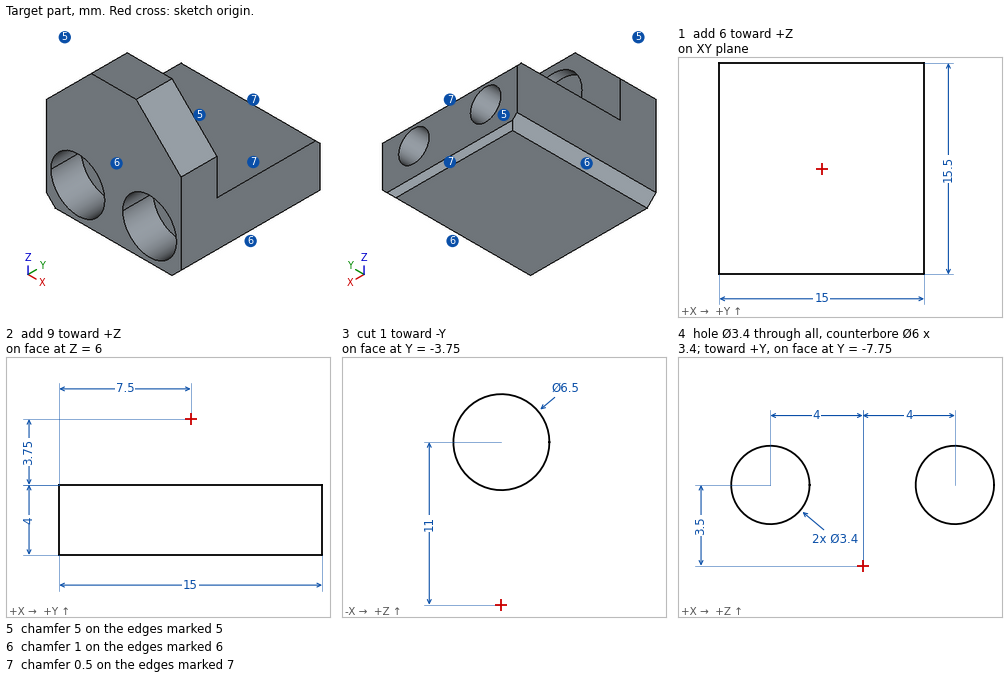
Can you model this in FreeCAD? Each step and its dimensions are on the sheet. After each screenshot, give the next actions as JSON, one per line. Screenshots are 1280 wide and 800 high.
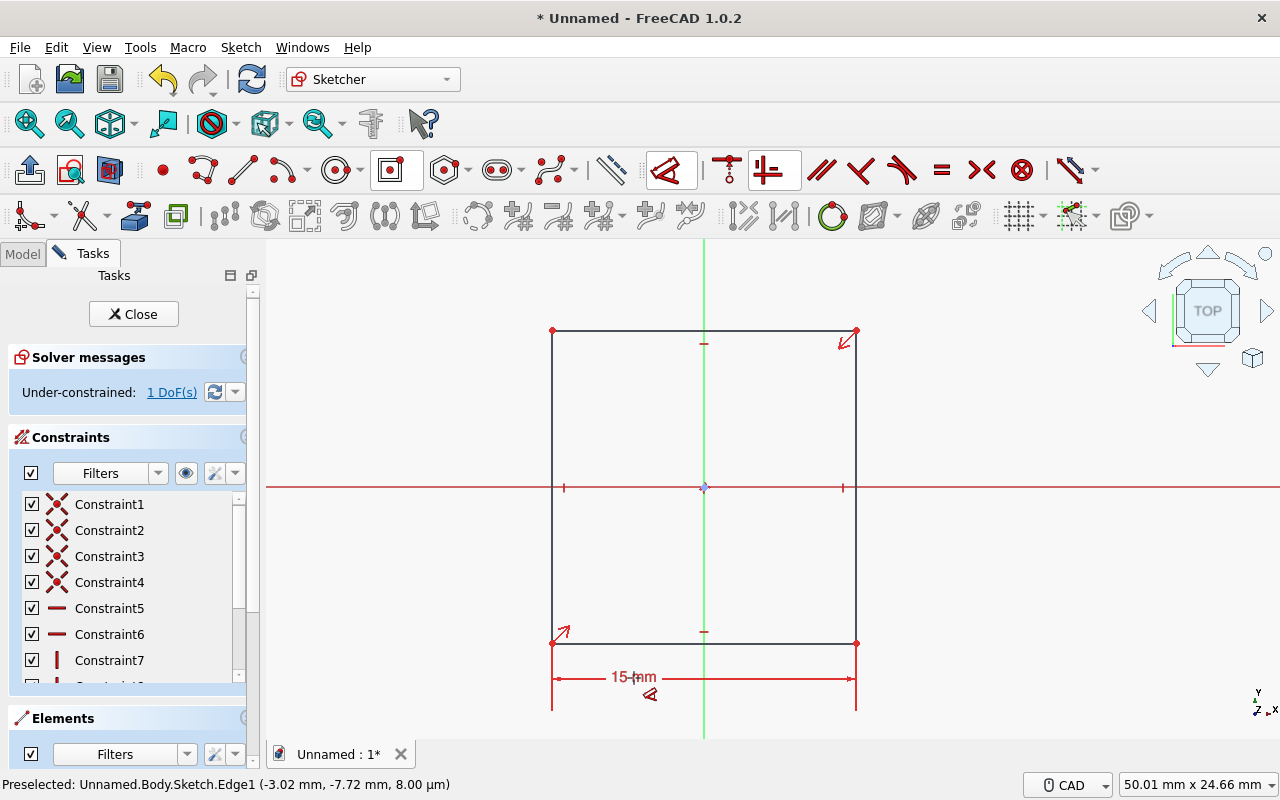
{"action": "left_click", "coordinate": [856, 550]}
{"action": "left_click", "coordinate": [890, 415]}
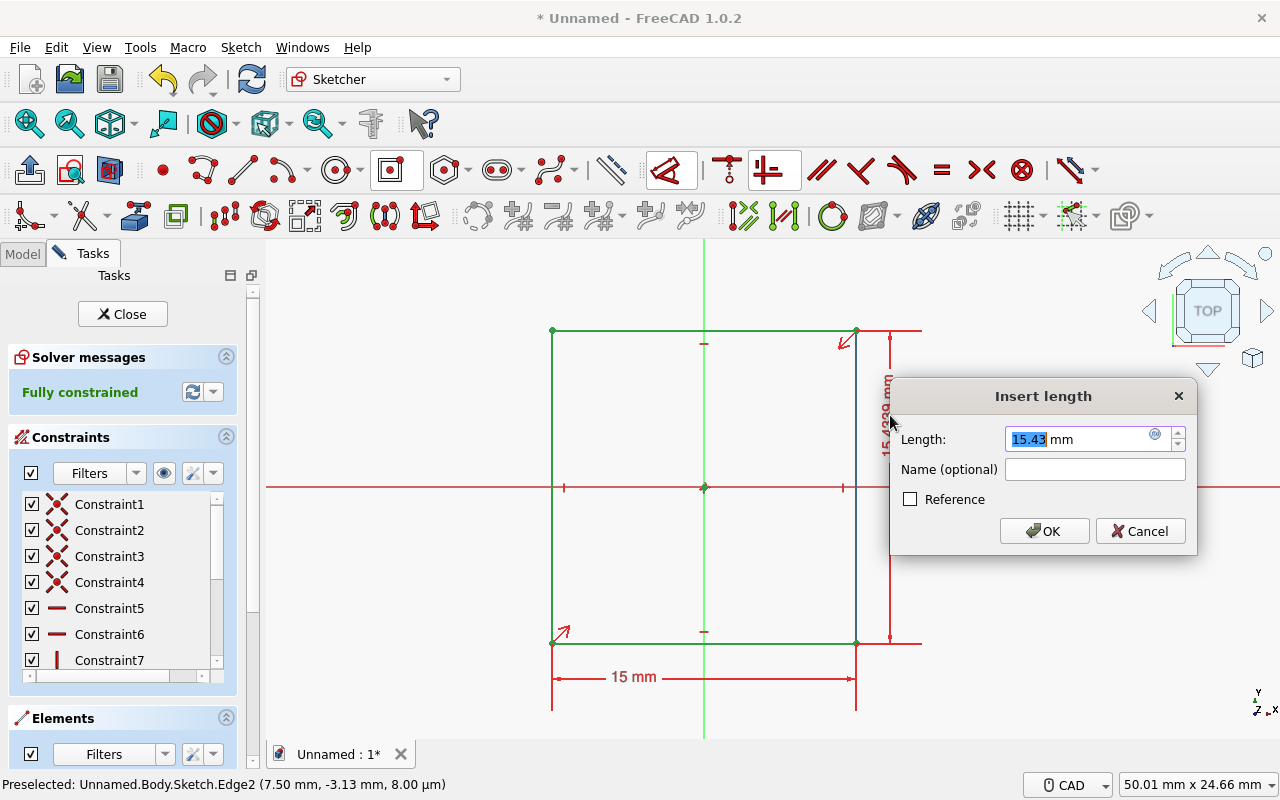
{"action": "type", "text": "15.5"}
{"action": "key", "text": "Return"}
{"action": "key", "text": "Escape"}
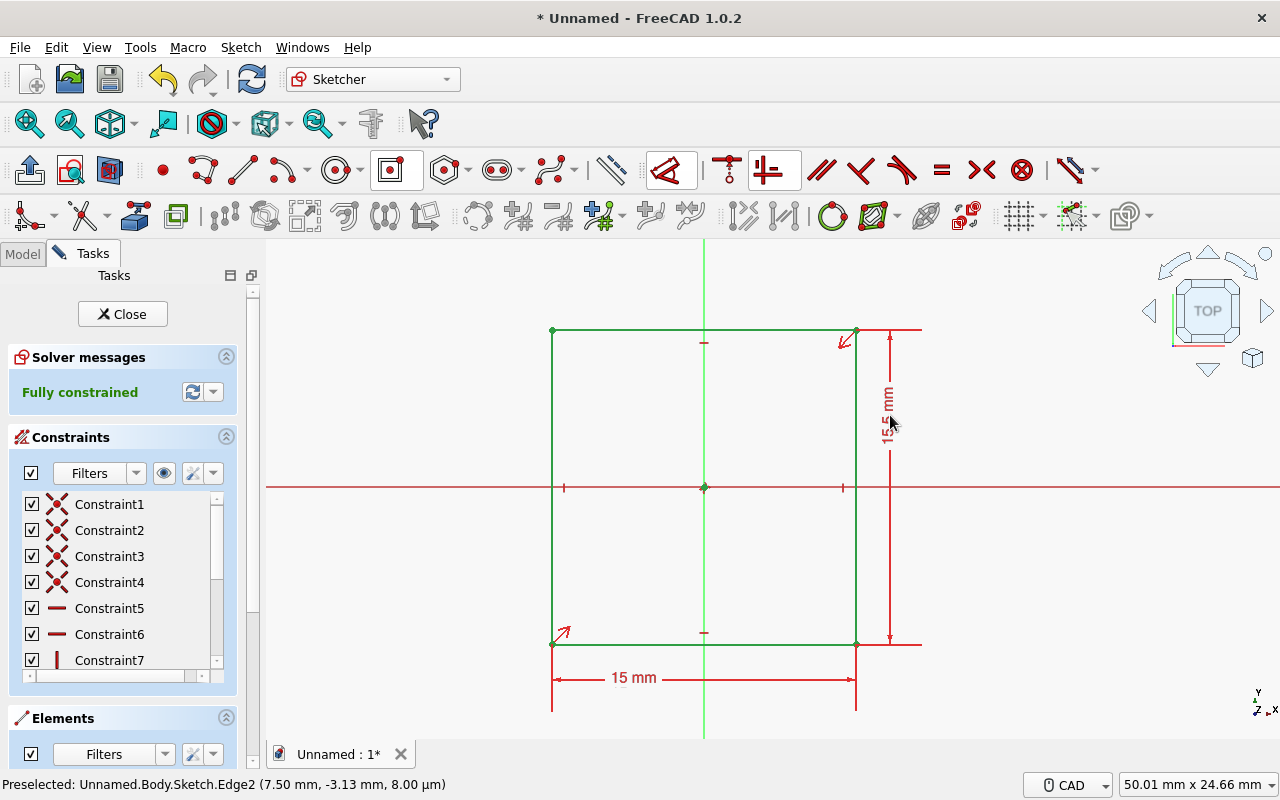
{"action": "left_click", "coordinate": [123, 314]}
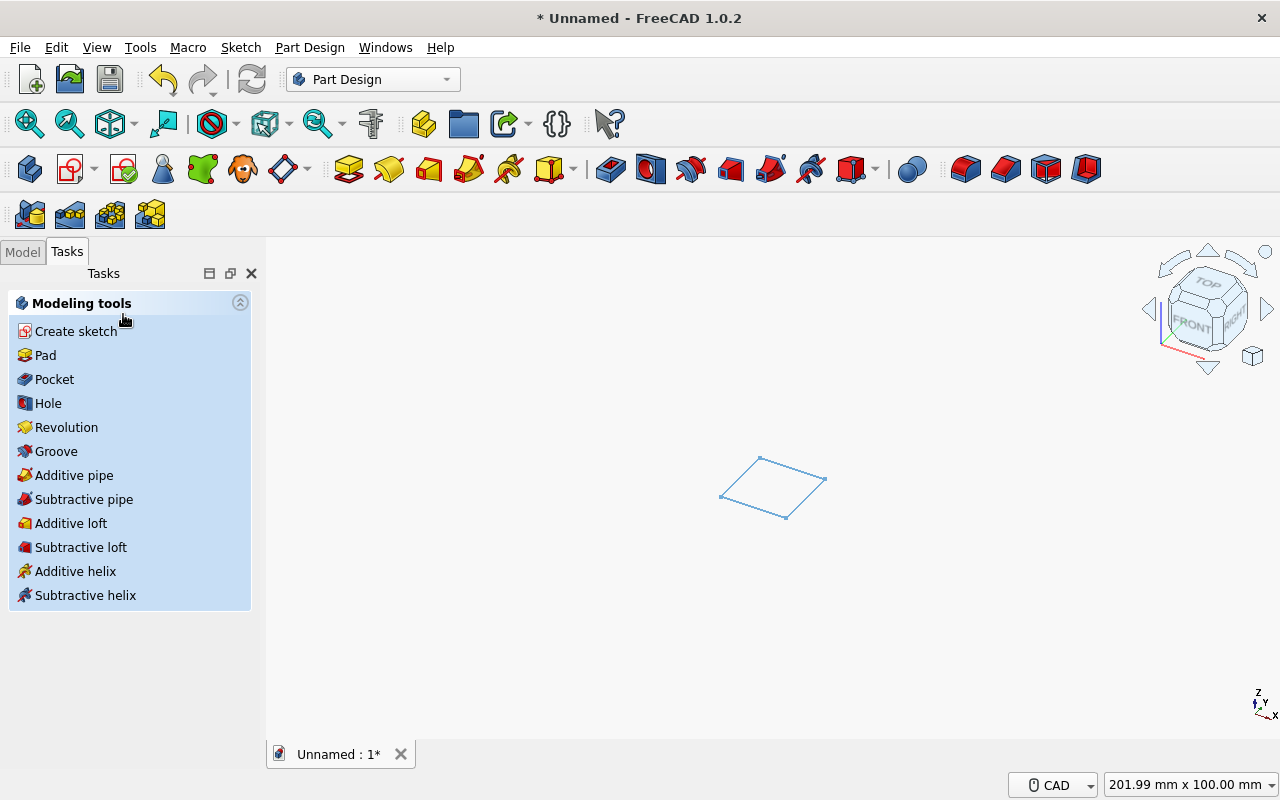
{"action": "left_click", "coordinate": [350, 170]}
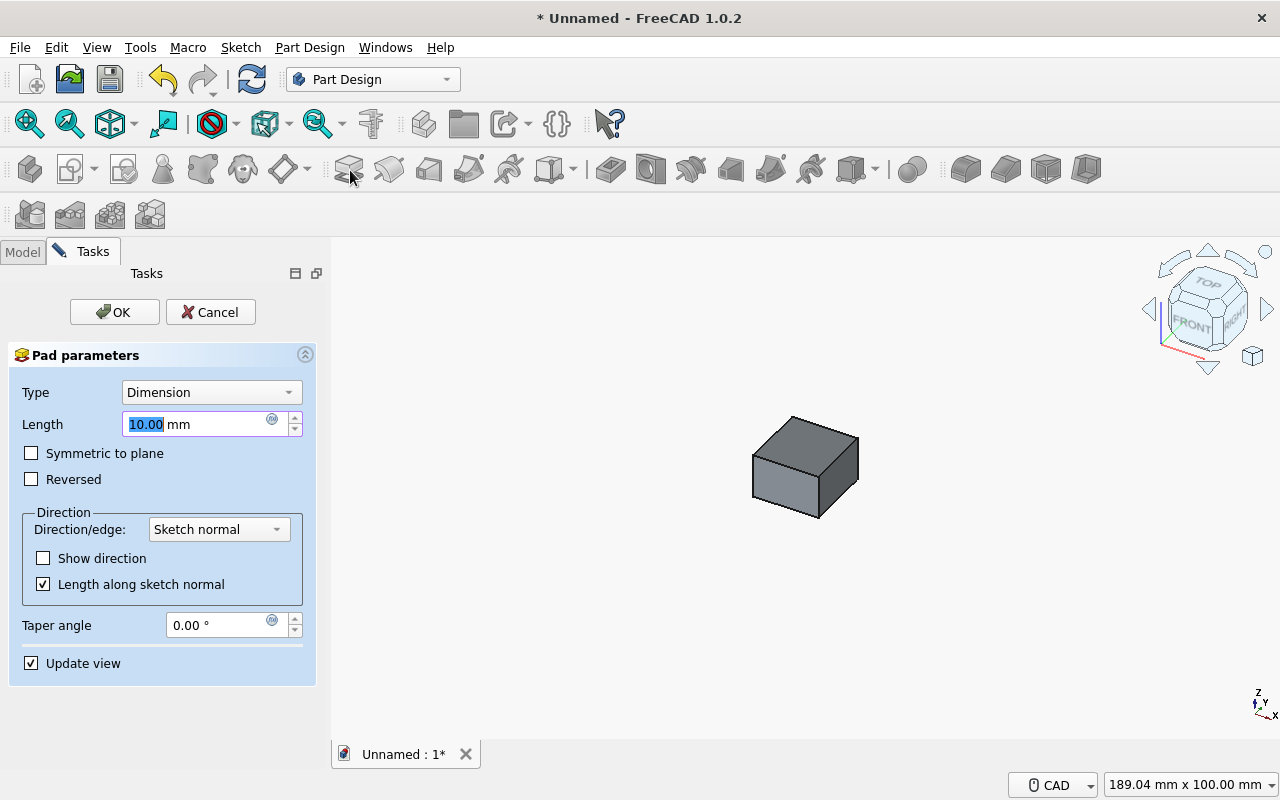
{"action": "type", "text": "6"}
{"action": "key", "text": "Tab"}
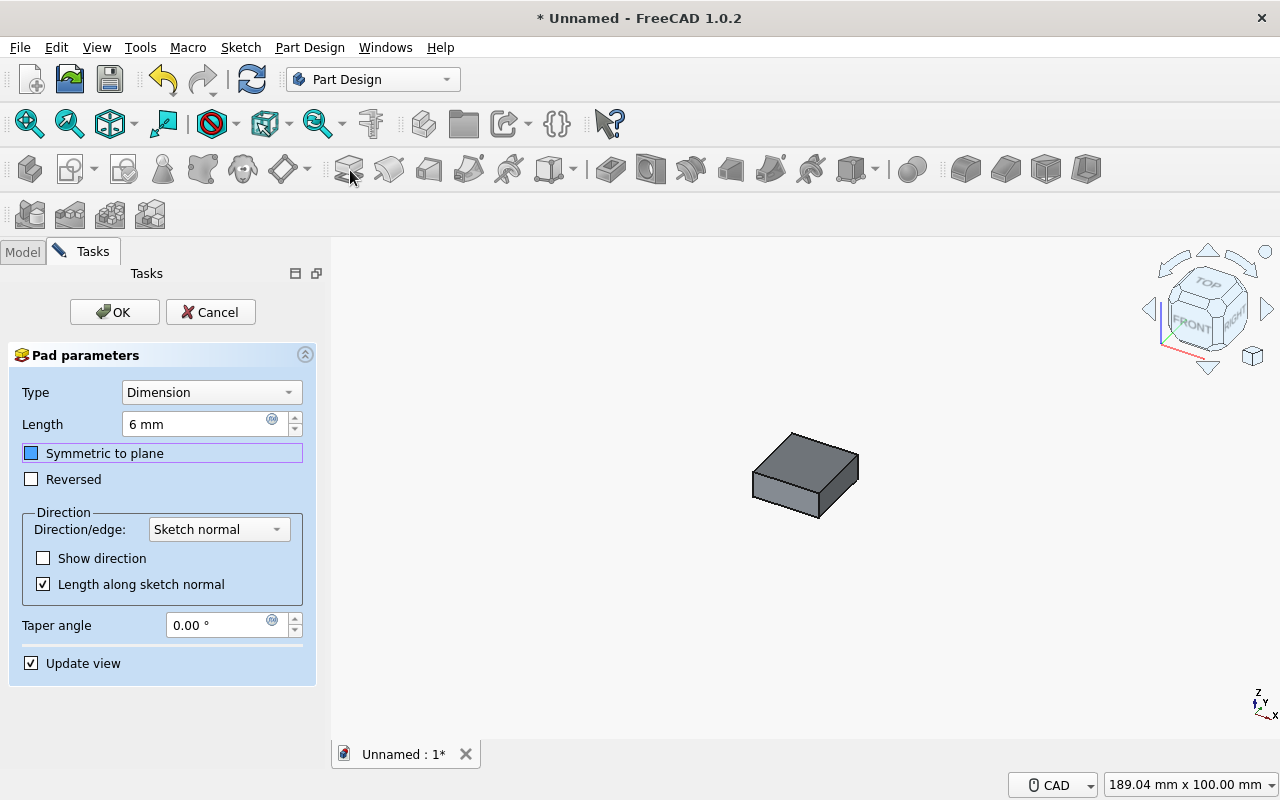
{"action": "left_click", "coordinate": [115, 312]}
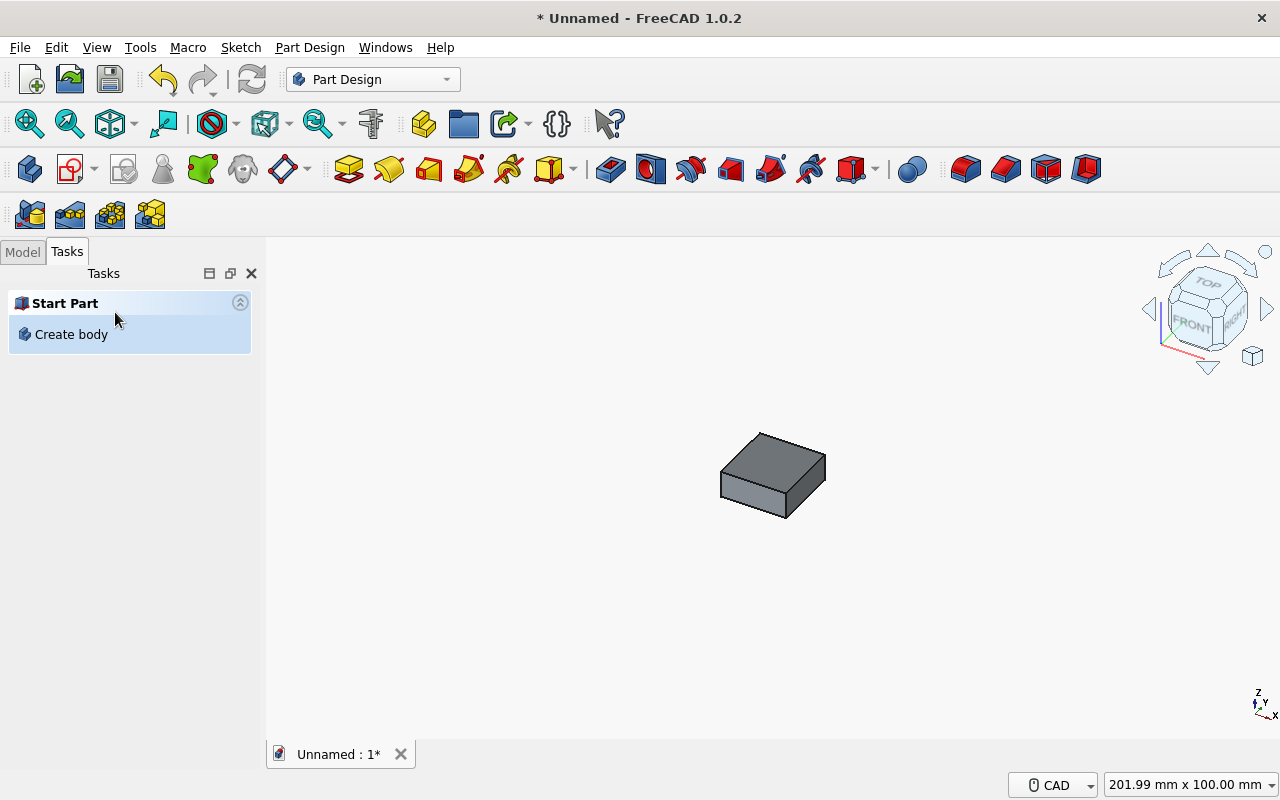
{"action": "key", "text": "v f"}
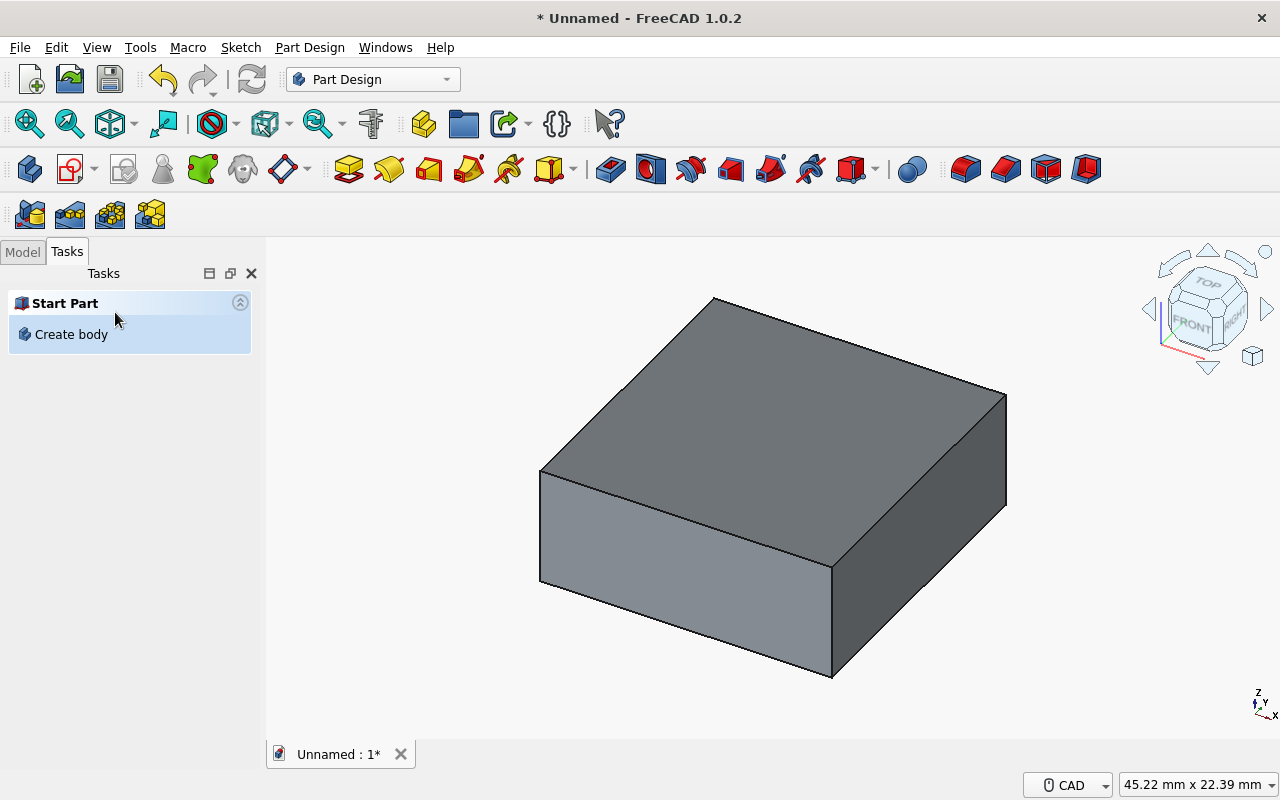
{"action": "left_click", "coordinate": [773, 432]}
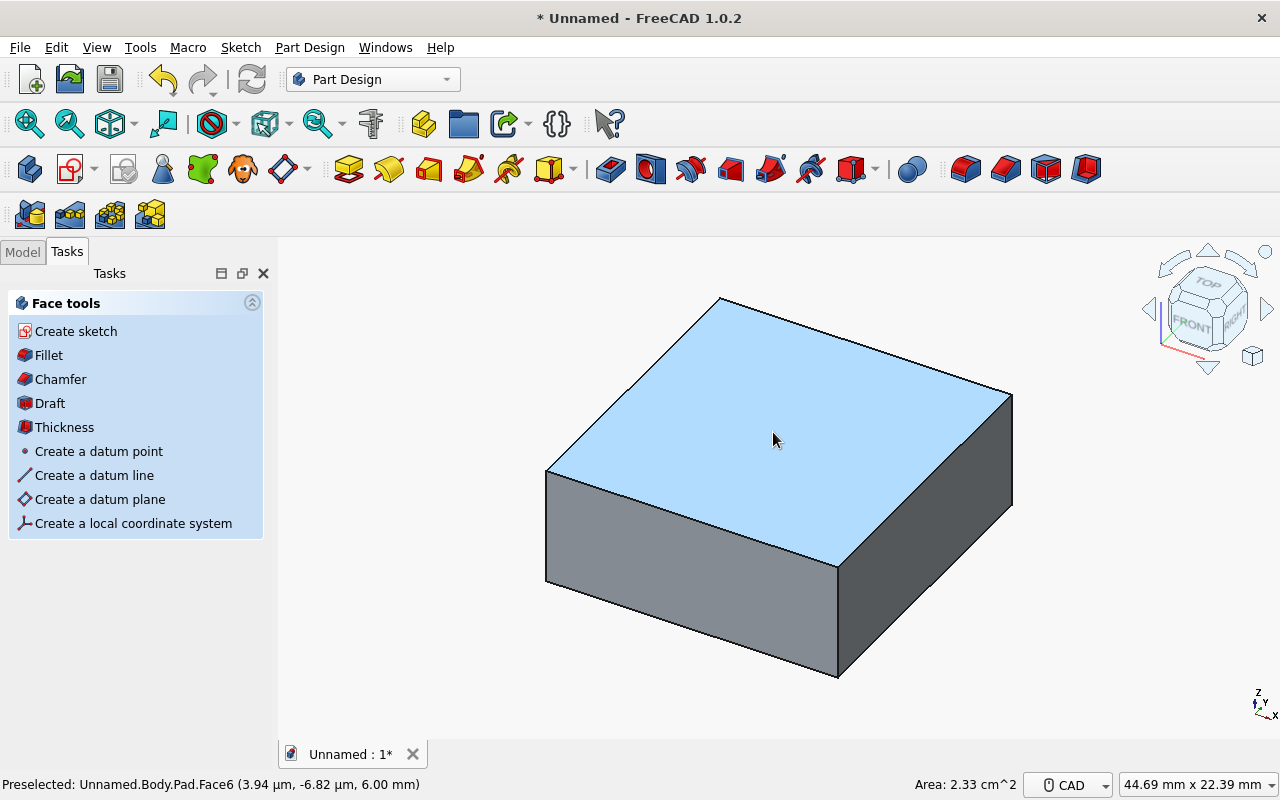
{"action": "left_click", "coordinate": [70, 170]}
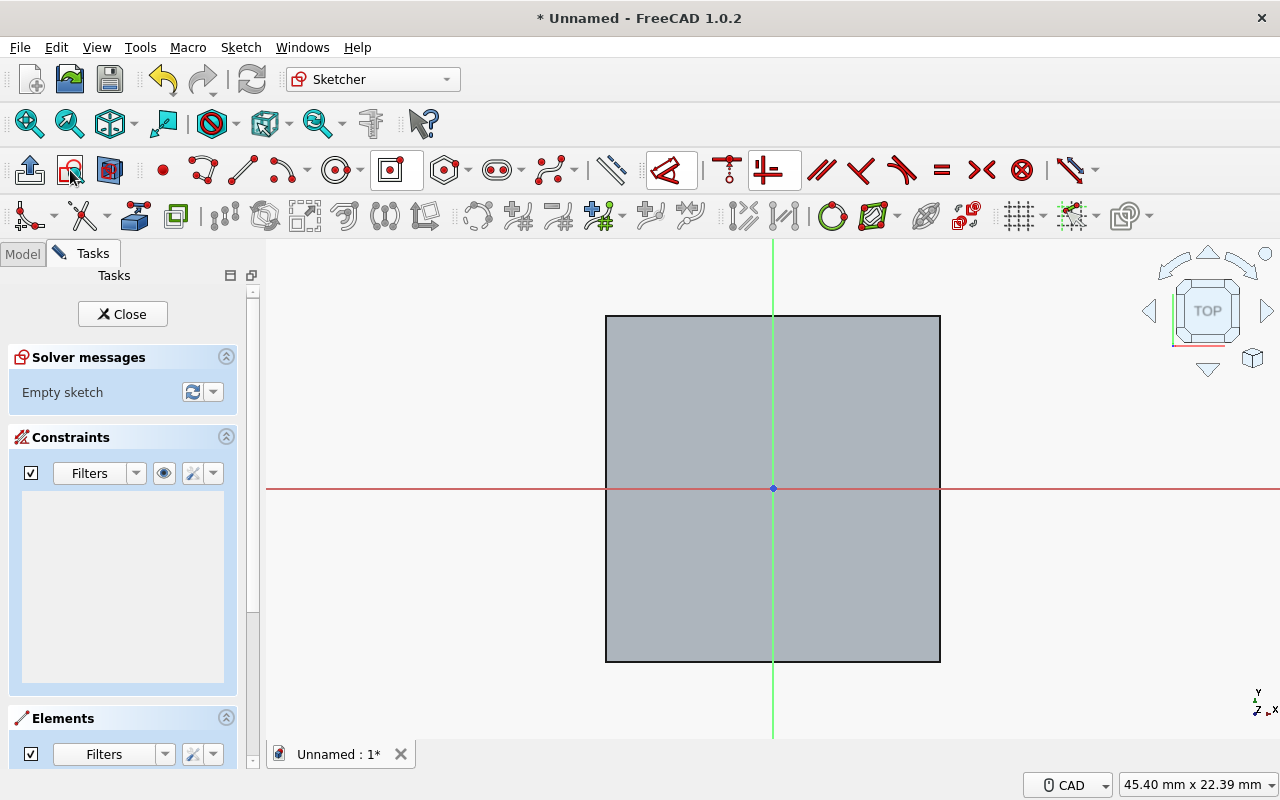
{"action": "scroll", "coordinate": [856, 681], "scroll_direction": "up", "scroll_amount": 3}